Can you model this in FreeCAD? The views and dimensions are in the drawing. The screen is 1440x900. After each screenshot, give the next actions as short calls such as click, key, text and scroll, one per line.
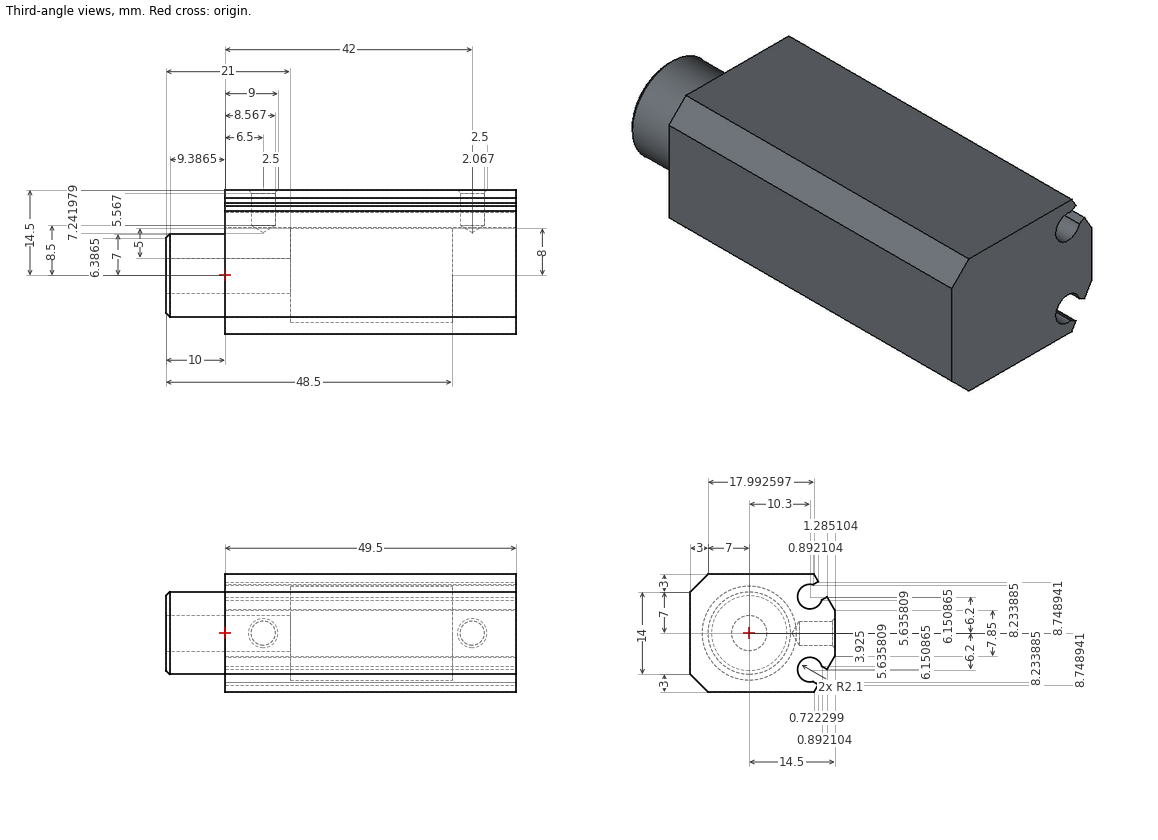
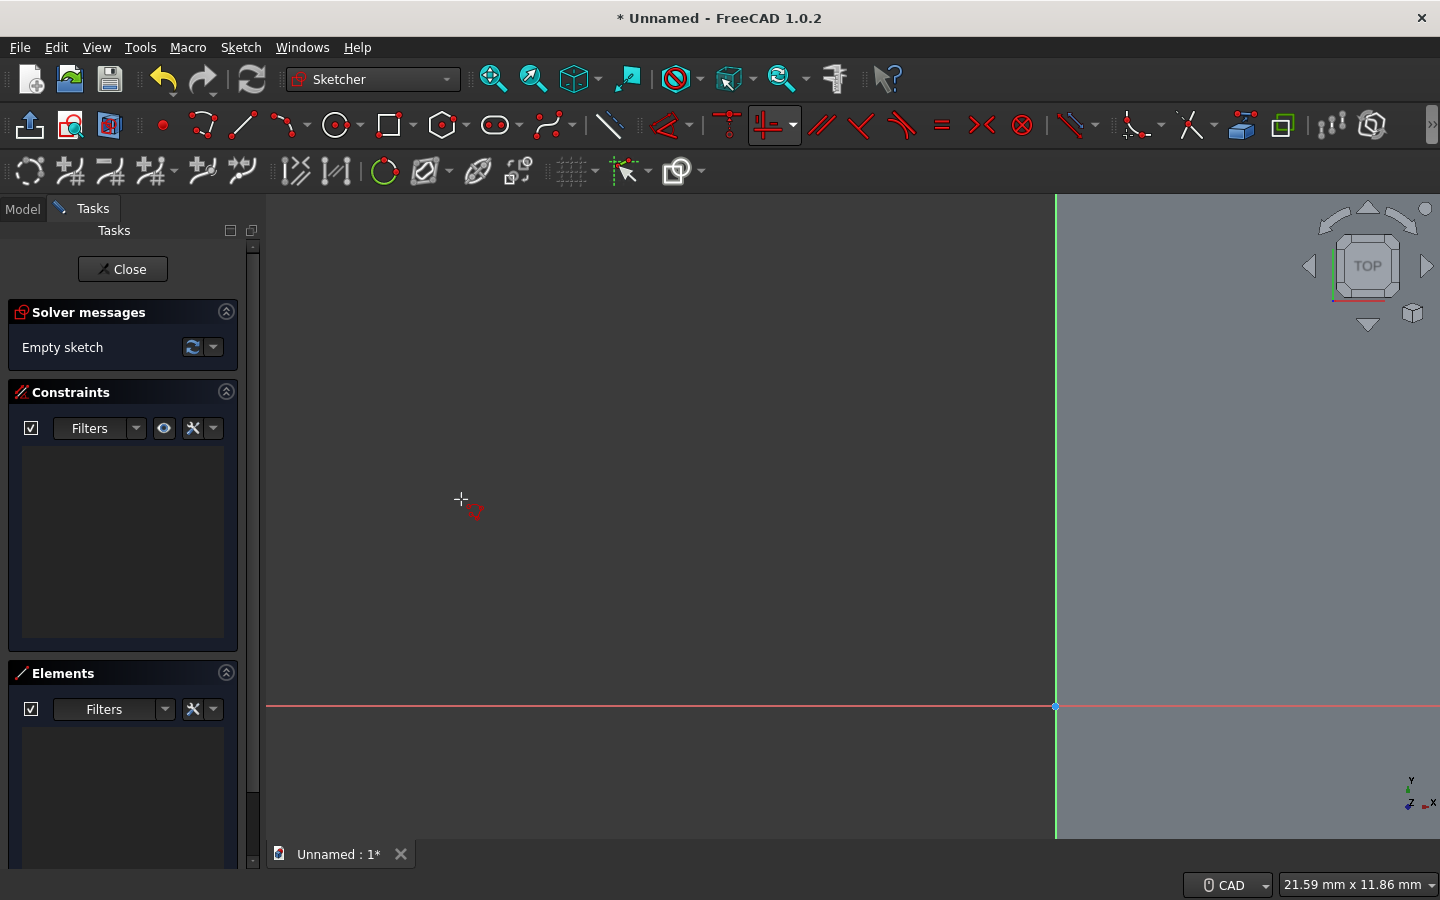
click(1056, 706)
click(1047, 325)
click(545, 325)
click(512, 359)
click(512, 697)
click(1056, 706)
key(Escape)
key(Escape)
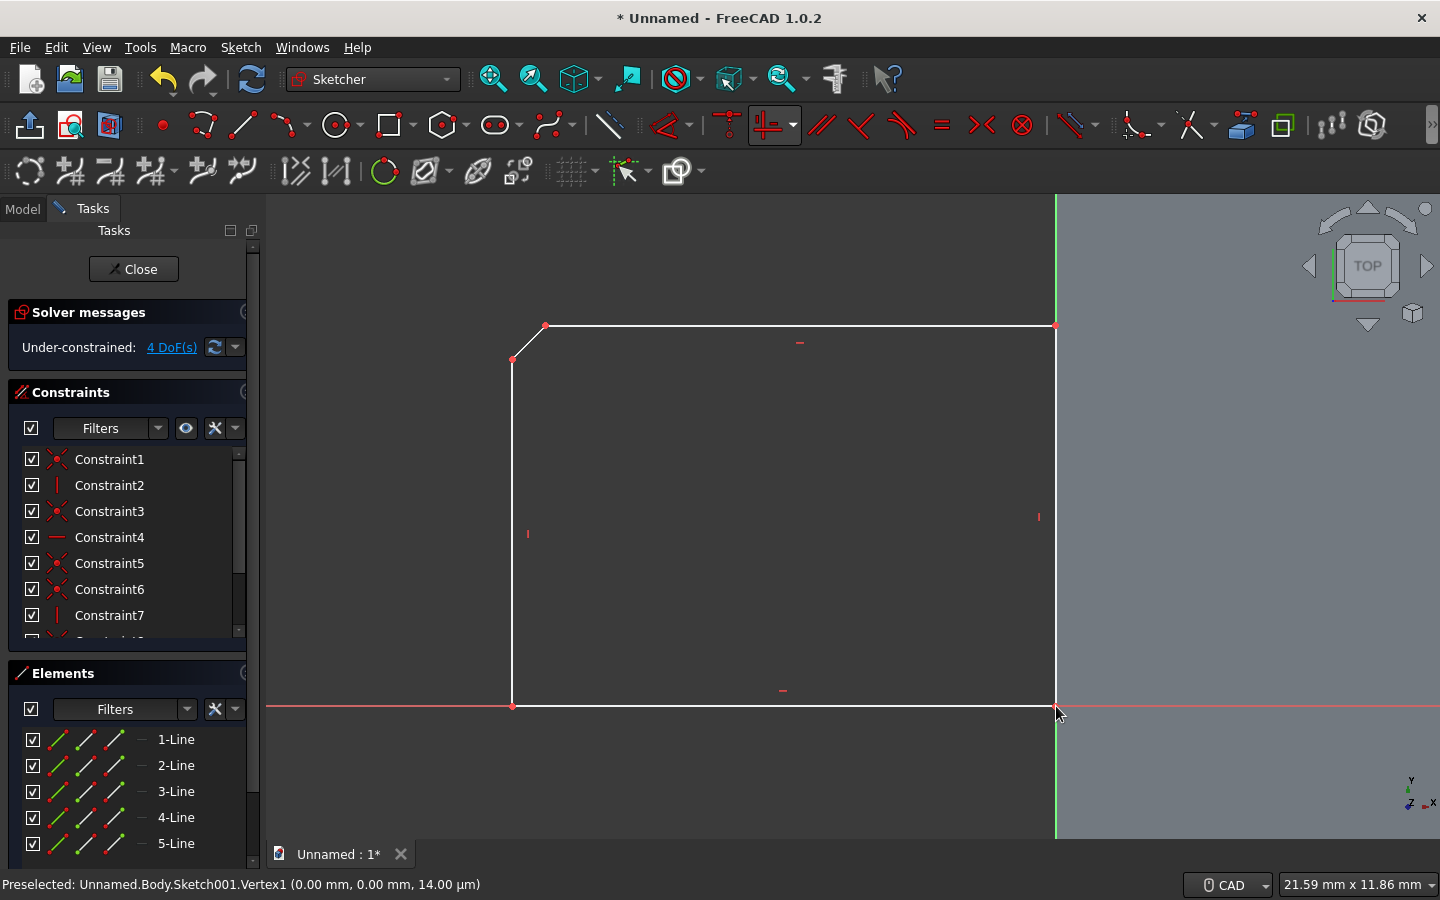
click(664, 126)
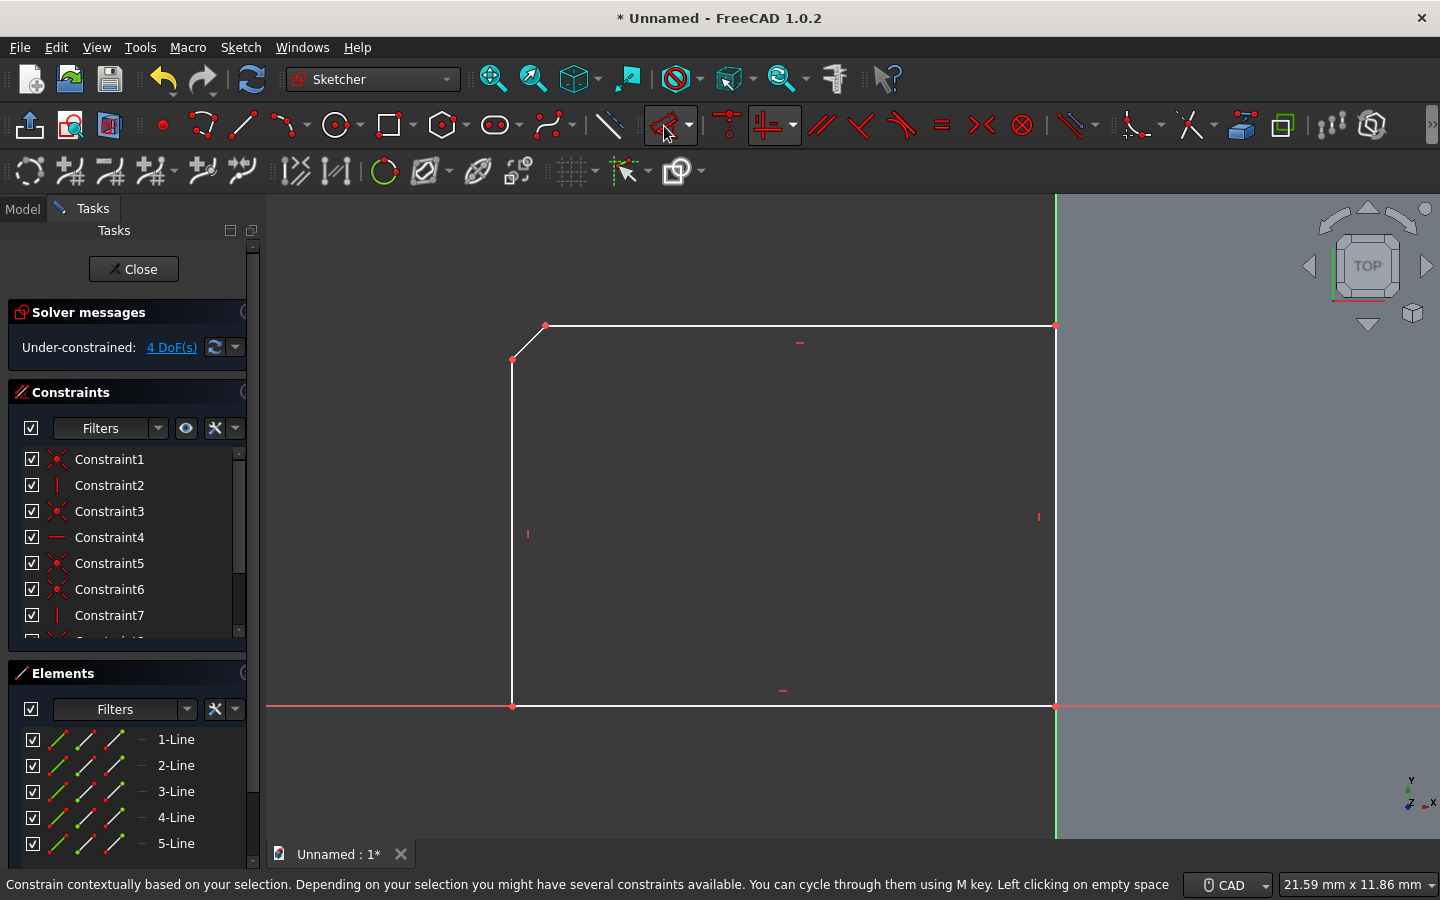
click(1056, 592)
click(1090, 516)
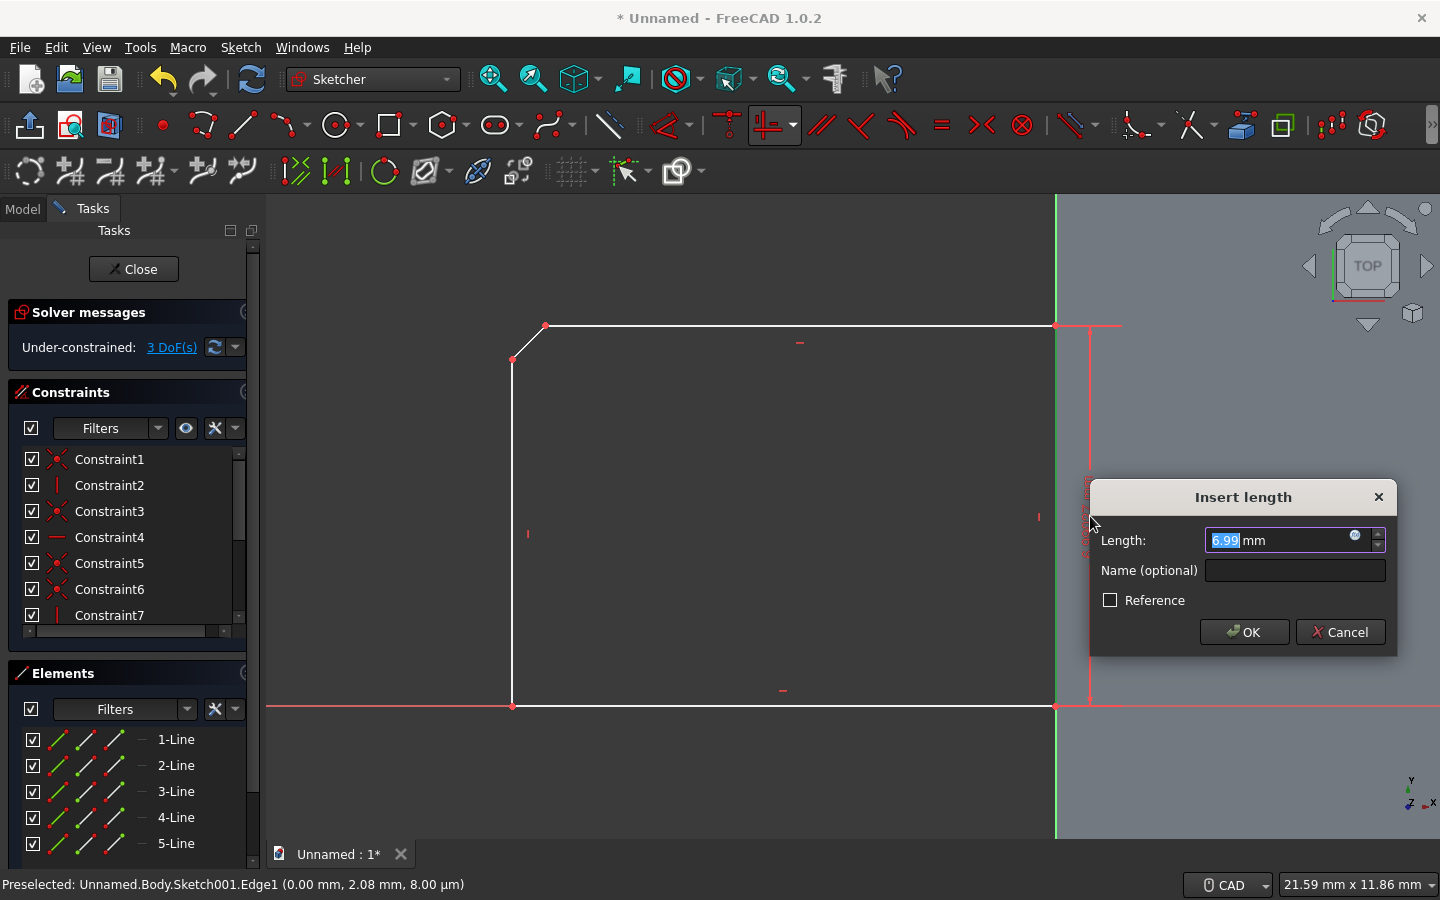
text(7)
key(Return)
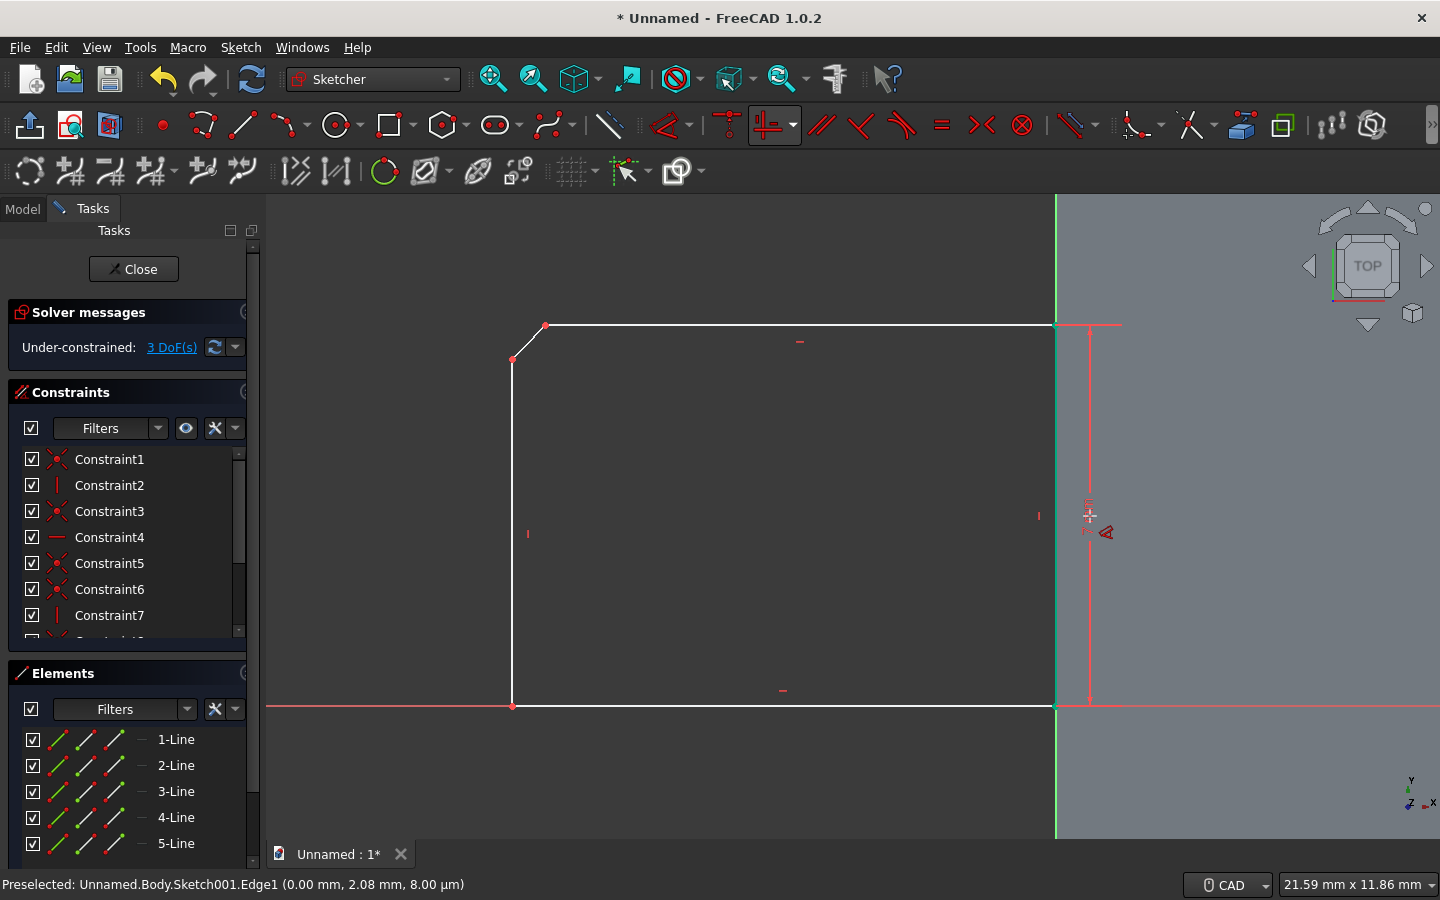
click(675, 706)
click(784, 740)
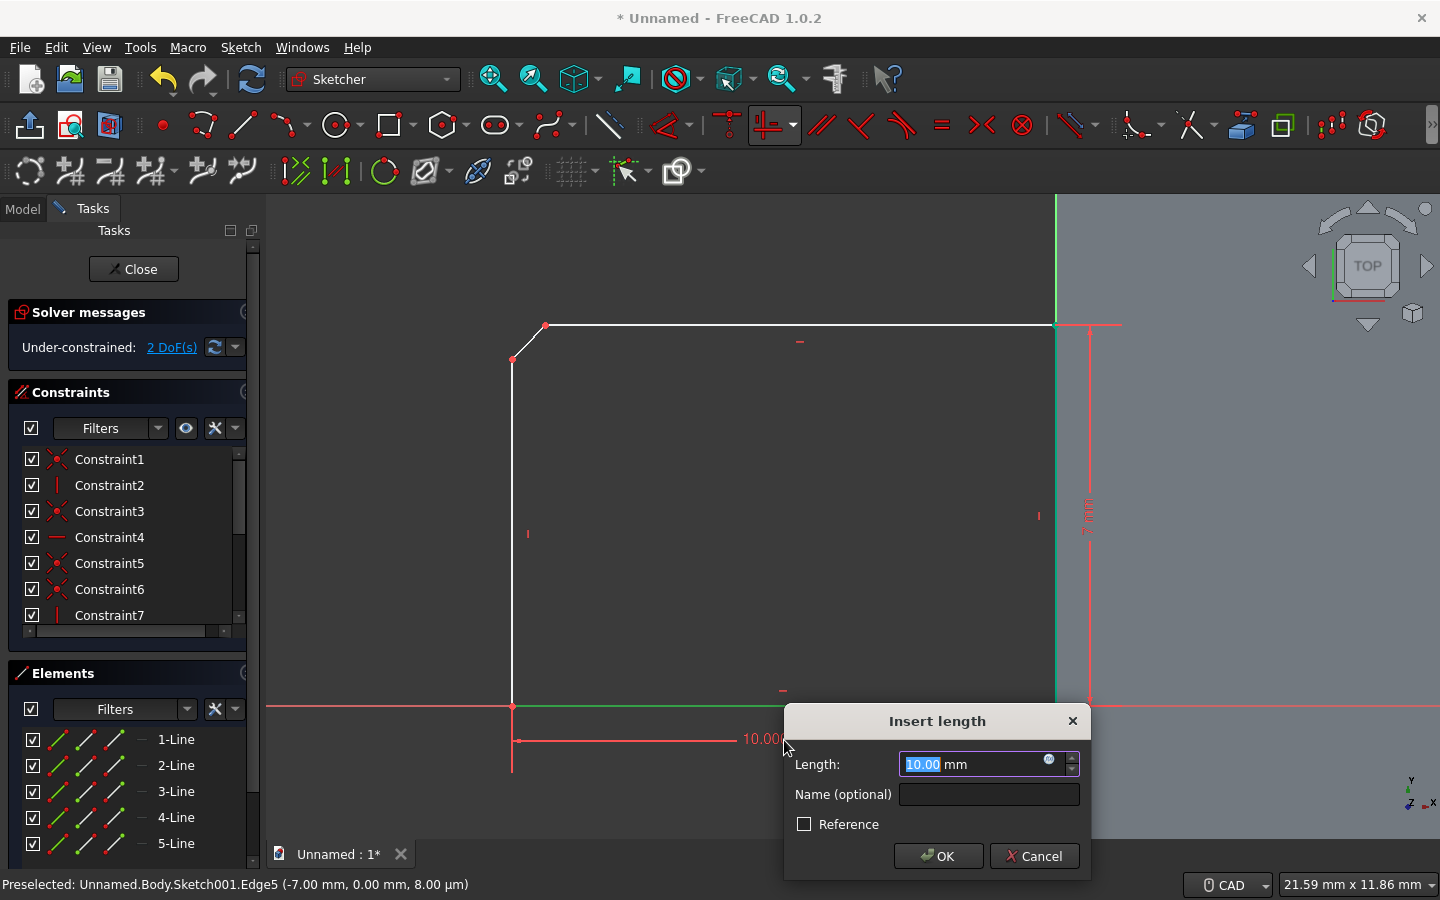
text(10)
key(Return)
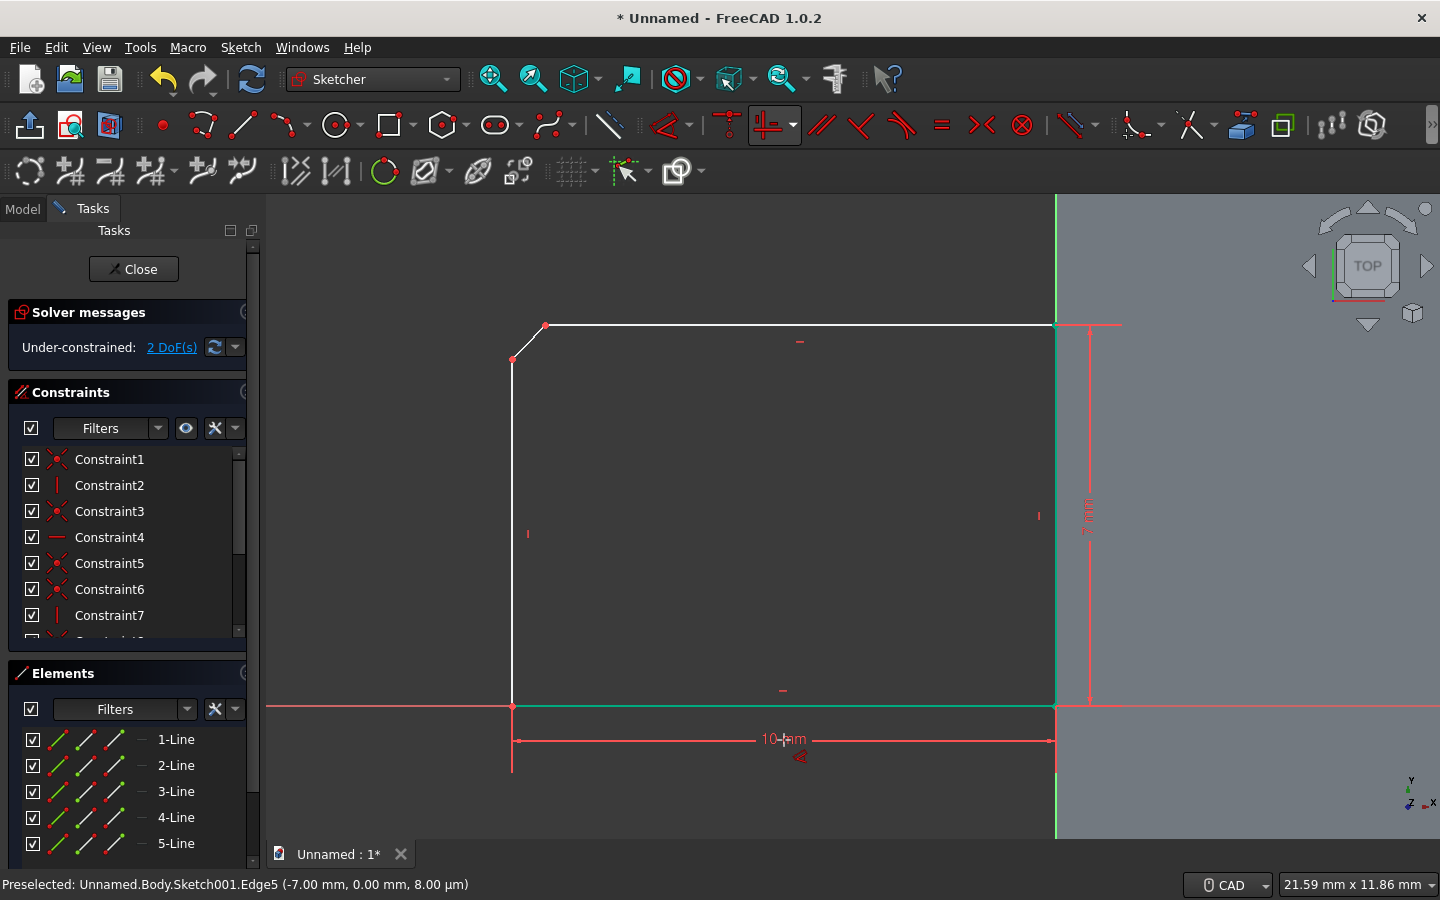
click(903, 325)
click(800, 291)